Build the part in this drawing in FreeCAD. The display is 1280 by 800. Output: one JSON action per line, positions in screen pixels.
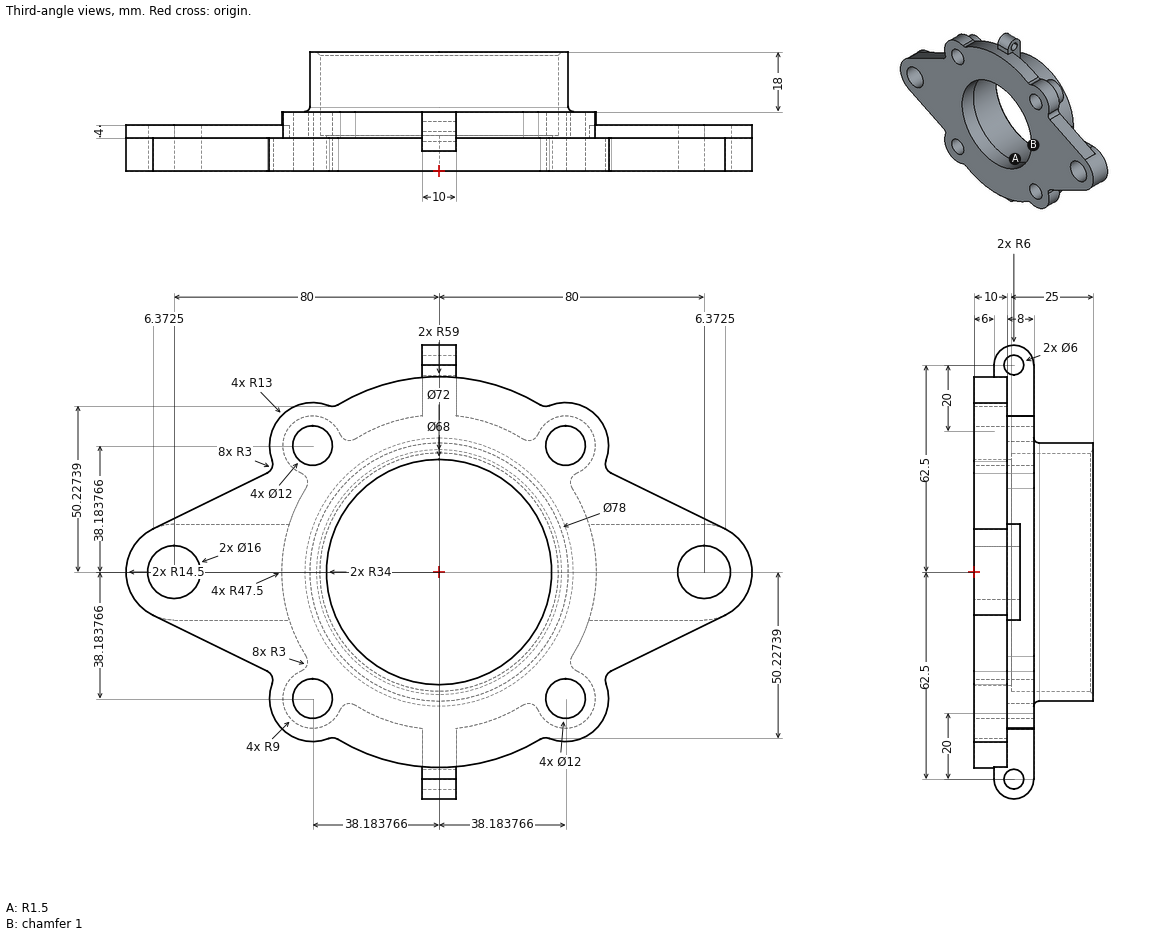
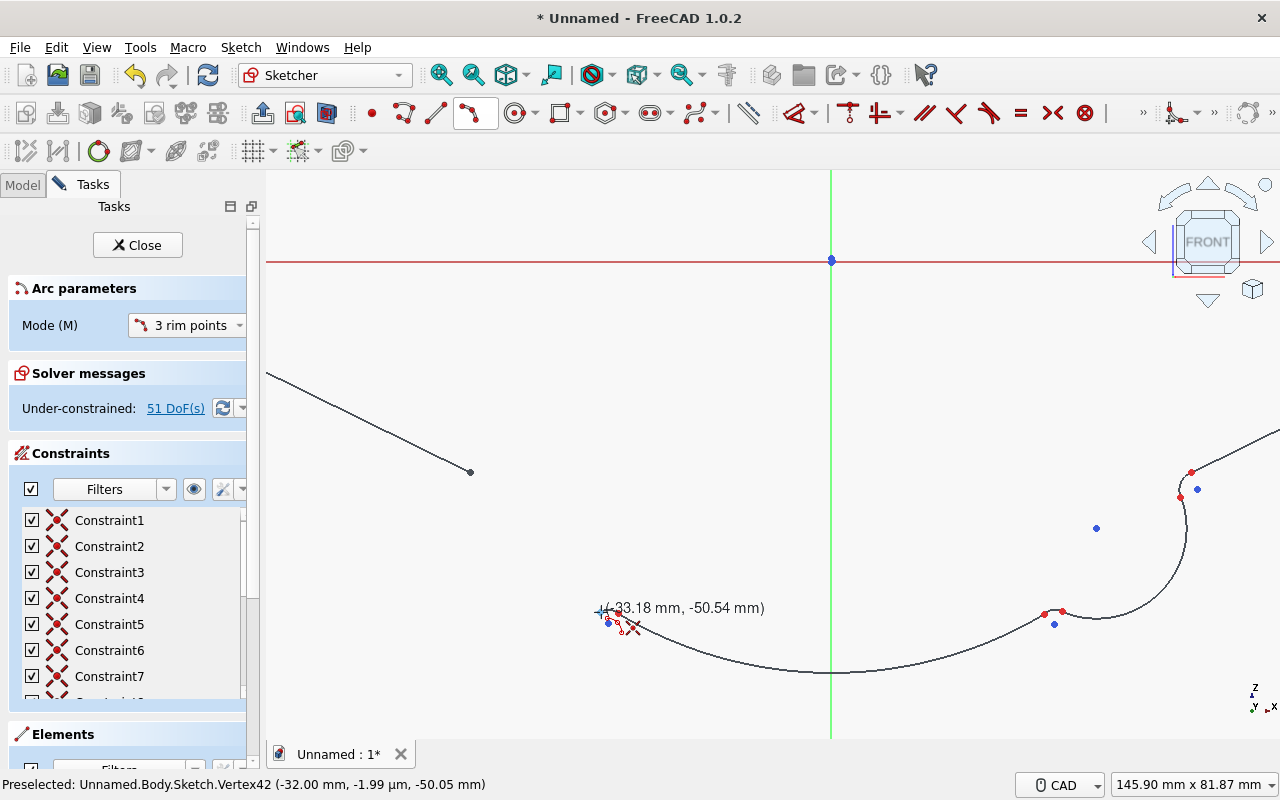
{"action": "left_click", "coordinate": [600, 613]}
{"action": "left_click", "coordinate": [481, 496]}
{"action": "left_click", "coordinate": [503, 592]}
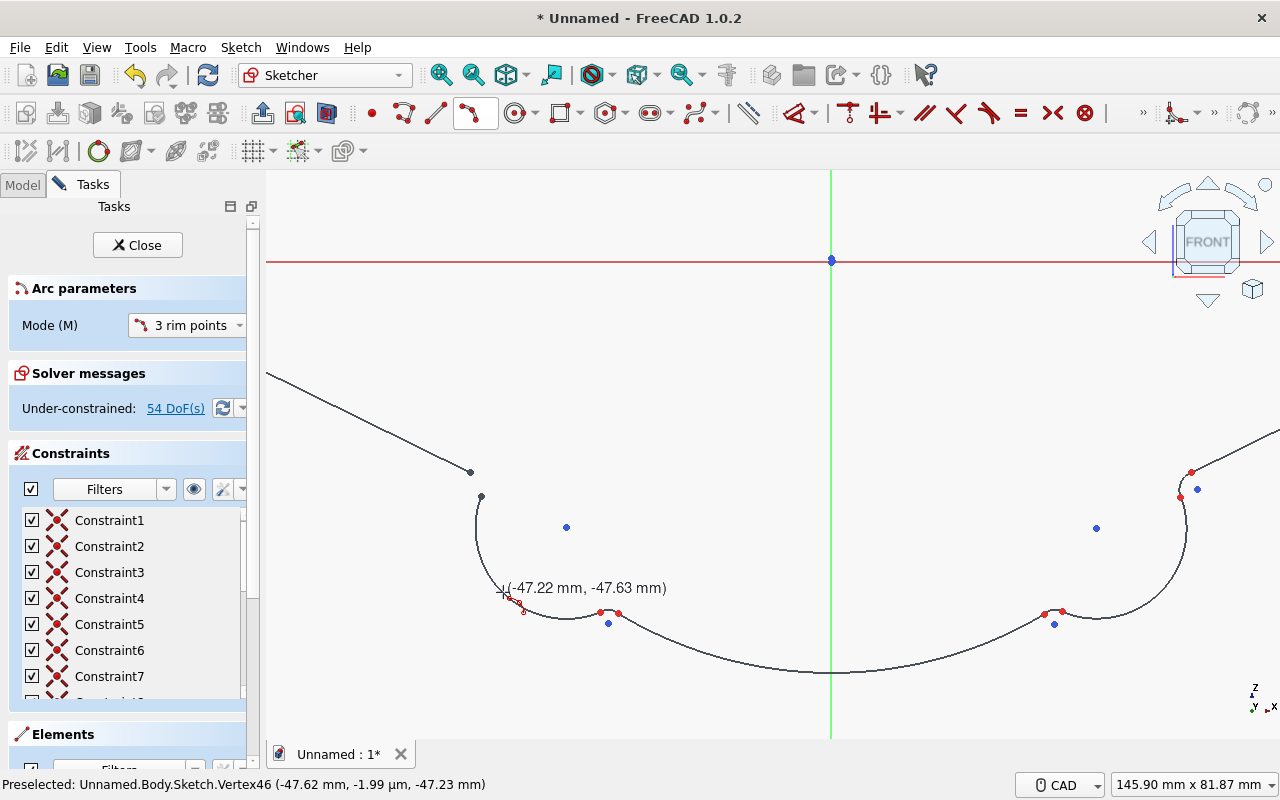
{"action": "left_click", "coordinate": [481, 497]}
{"action": "left_click", "coordinate": [471, 473]}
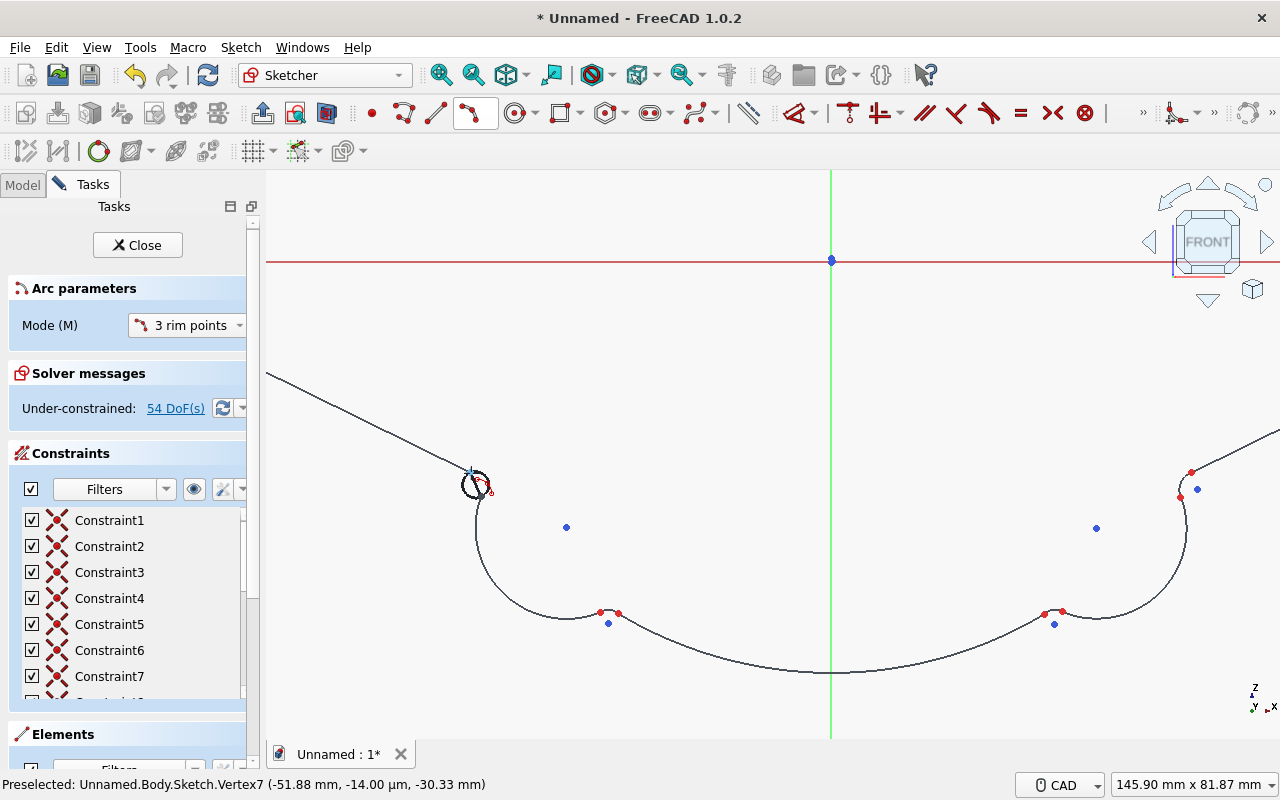
{"action": "scroll", "coordinate": [481, 481], "scroll_direction": "up", "scroll_amount": 6}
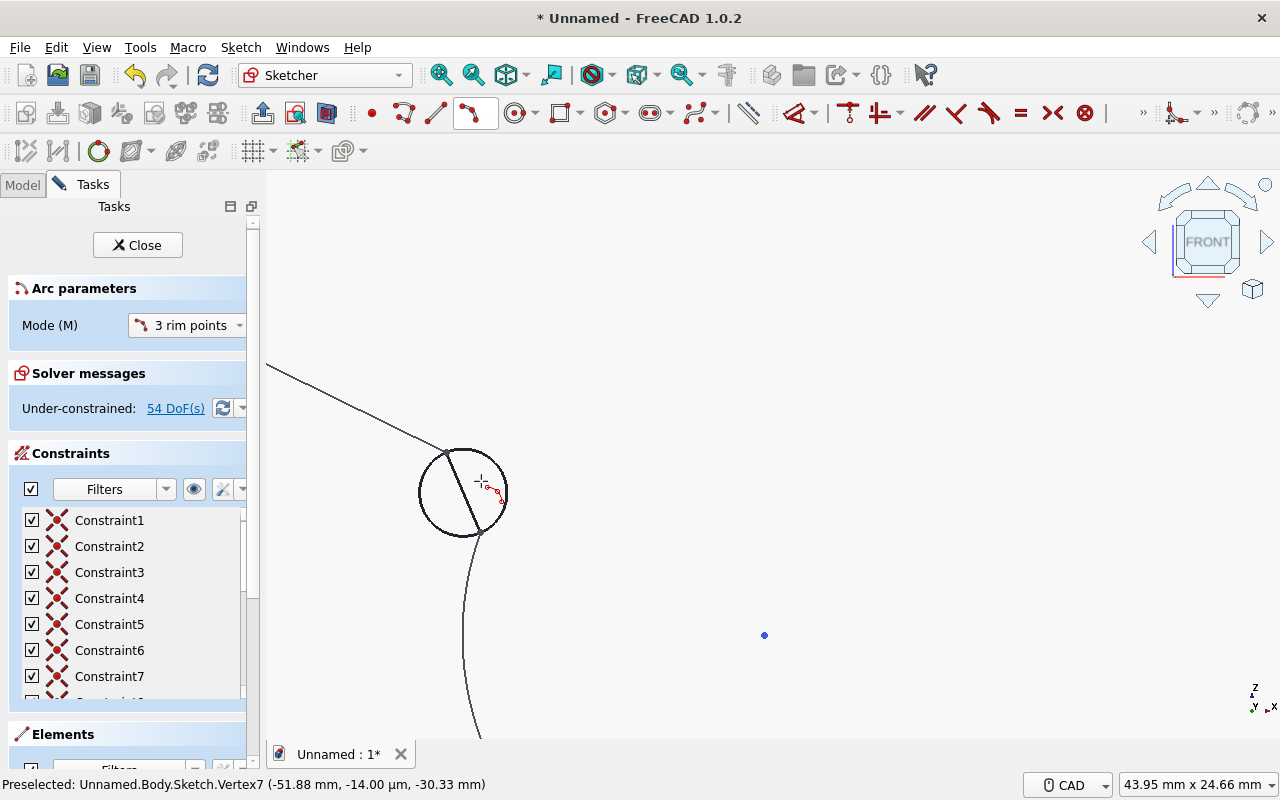
{"action": "left_click", "coordinate": [480, 479]}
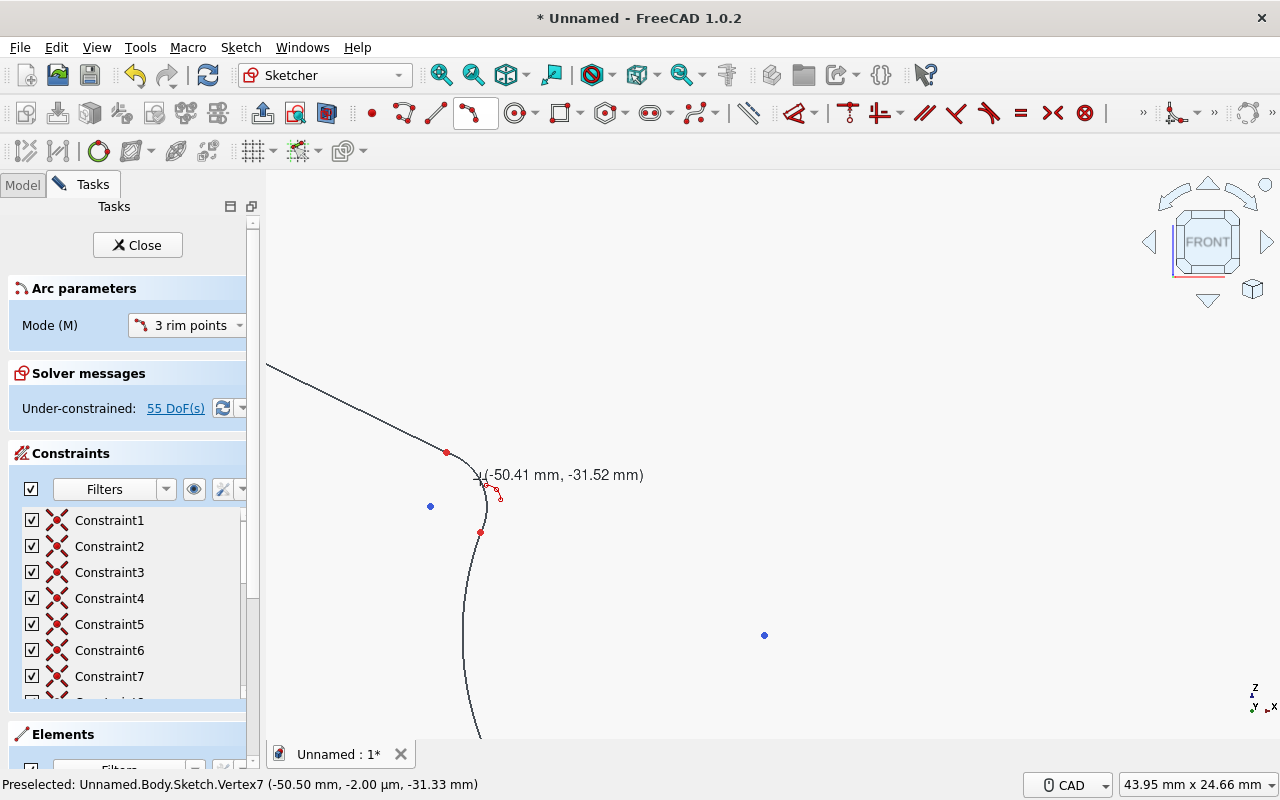
{"action": "scroll", "coordinate": [558, 564], "scroll_direction": "down", "scroll_amount": 10}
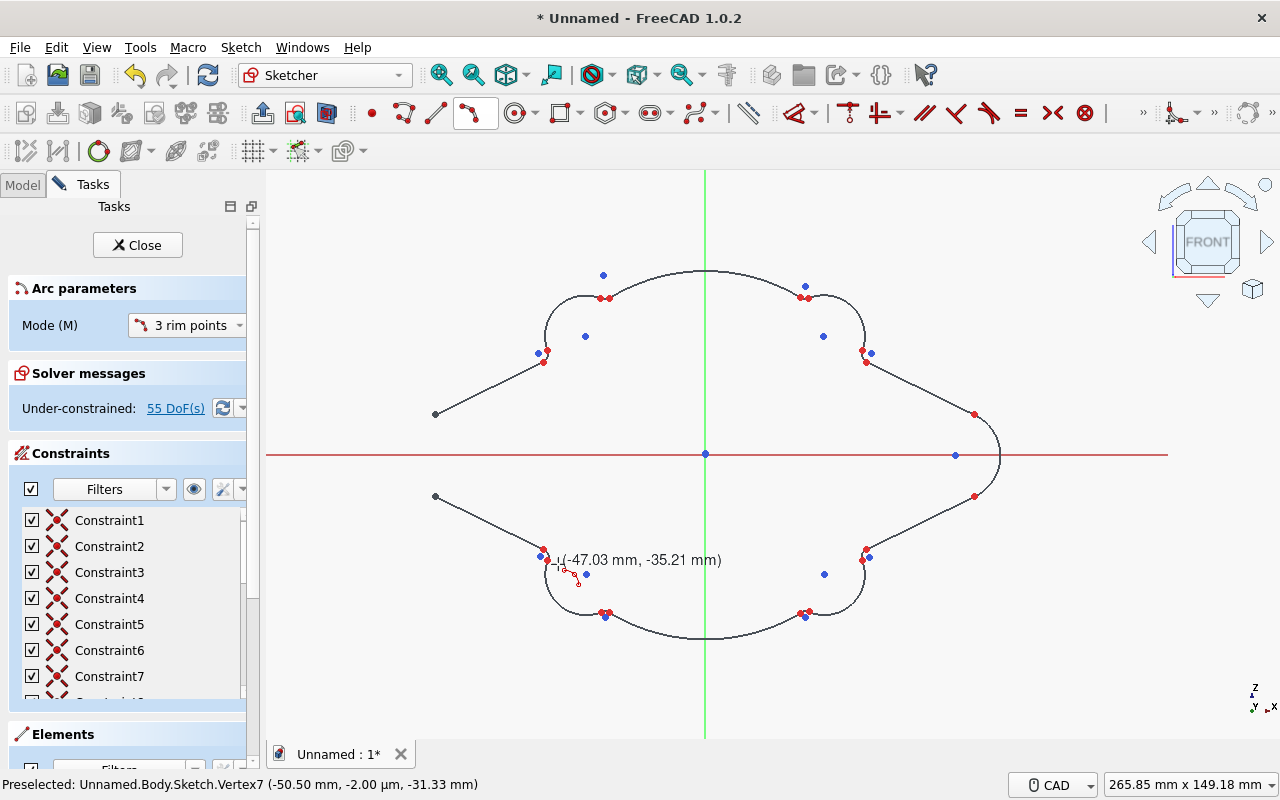
{"action": "left_click", "coordinate": [435, 497]}
{"action": "left_click", "coordinate": [435, 415]}
{"action": "left_click", "coordinate": [414, 435]}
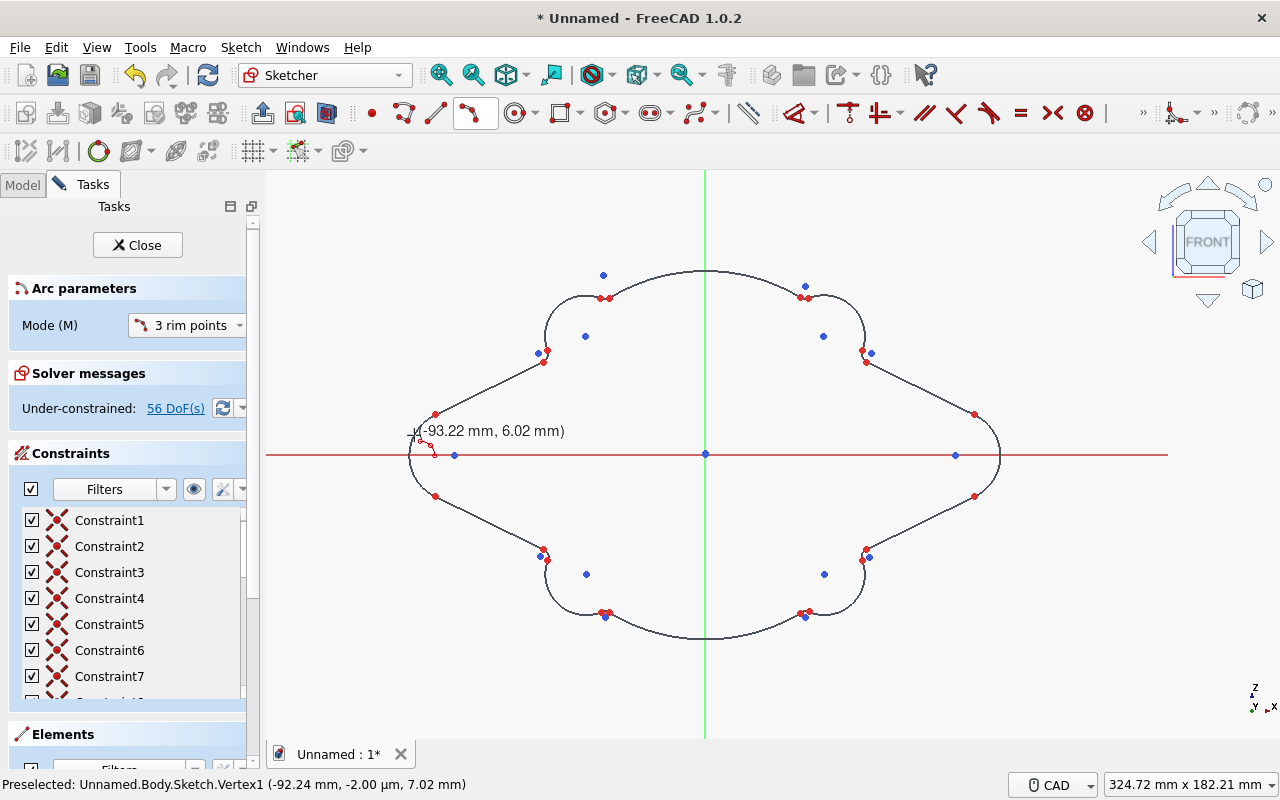
{"action": "left_click", "coordinate": [516, 114]}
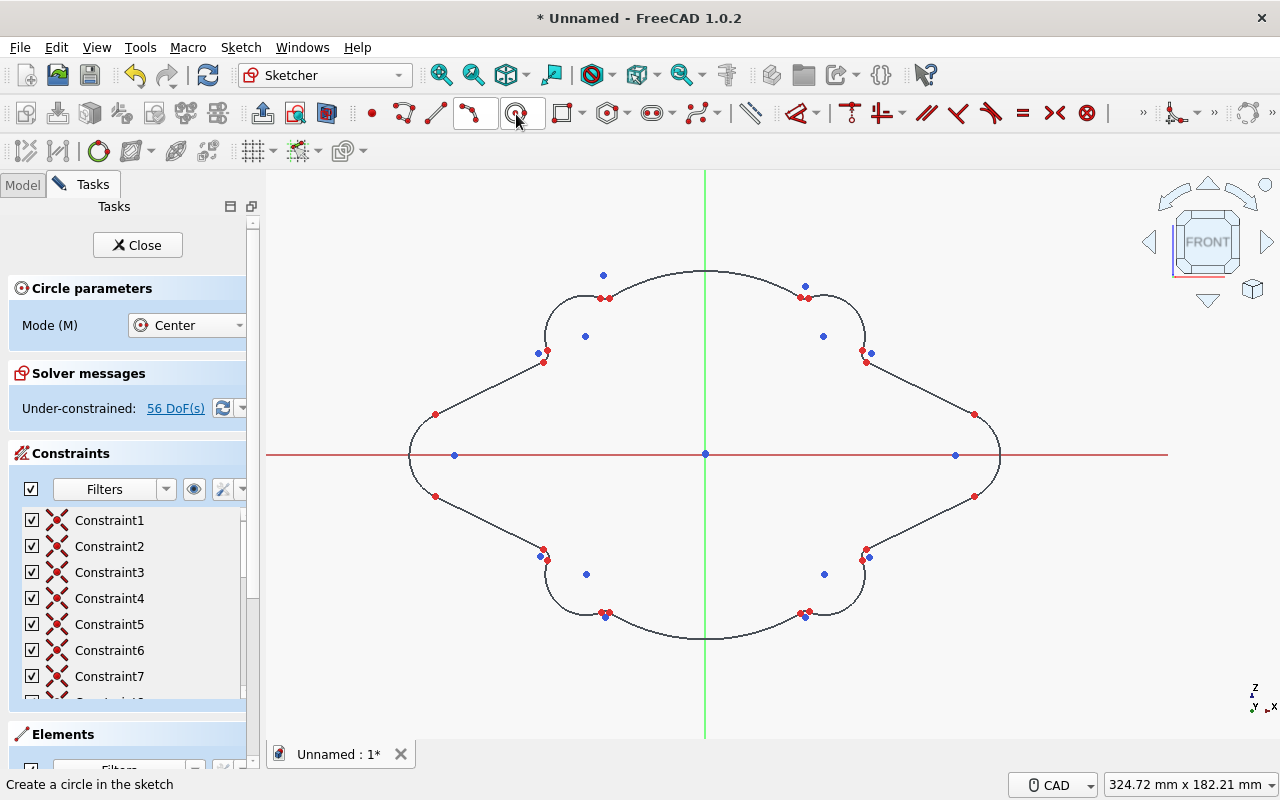
{"action": "left_click", "coordinate": [455, 455]}
{"action": "mouse_move", "coordinate": [473, 437]}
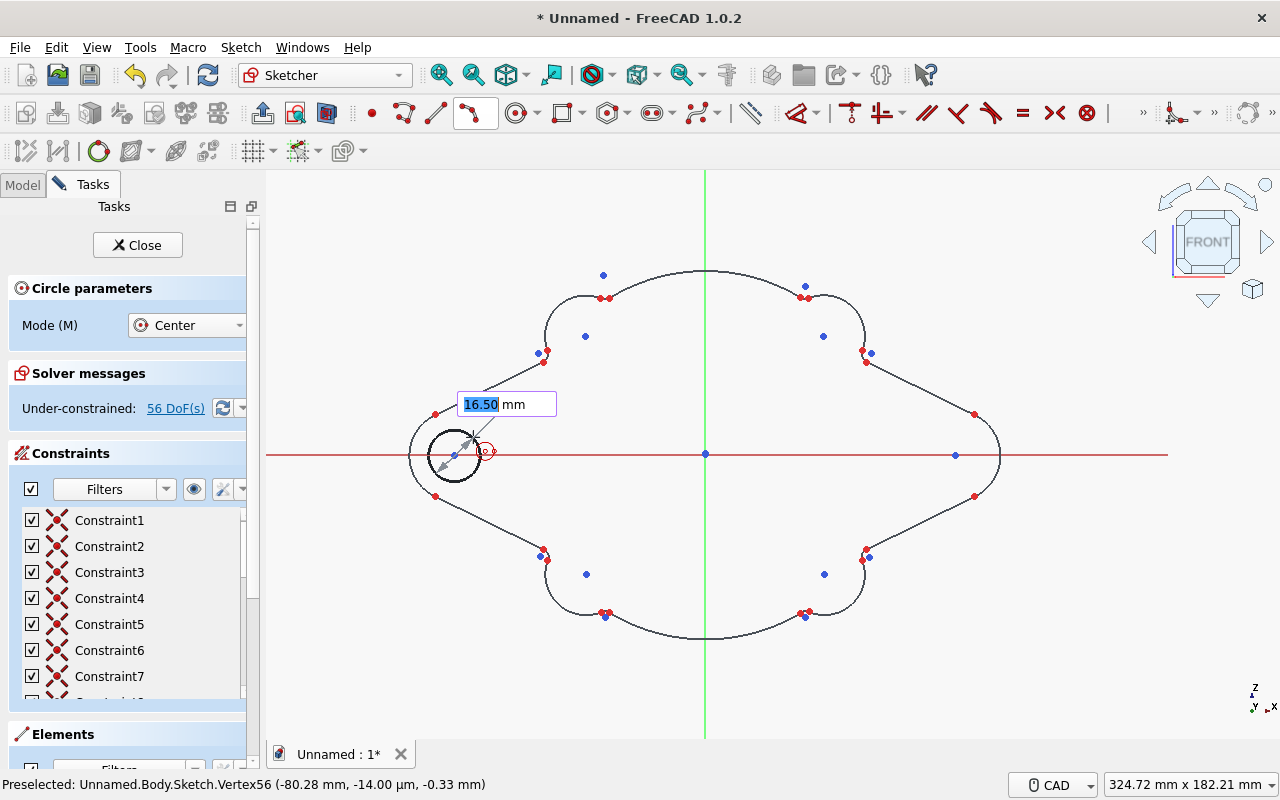
{"action": "type", "text": "16"}
{"action": "key", "text": "Return"}